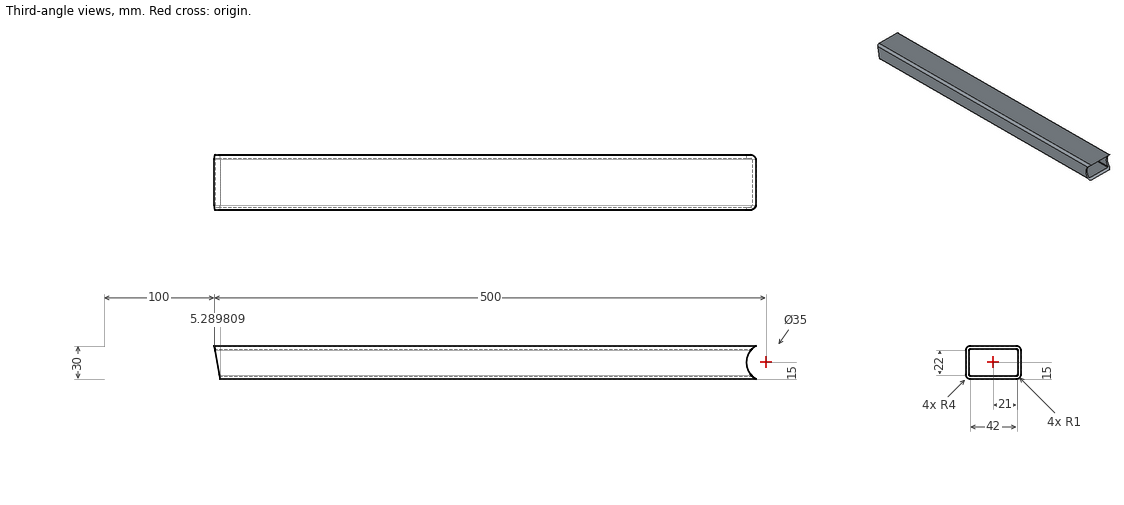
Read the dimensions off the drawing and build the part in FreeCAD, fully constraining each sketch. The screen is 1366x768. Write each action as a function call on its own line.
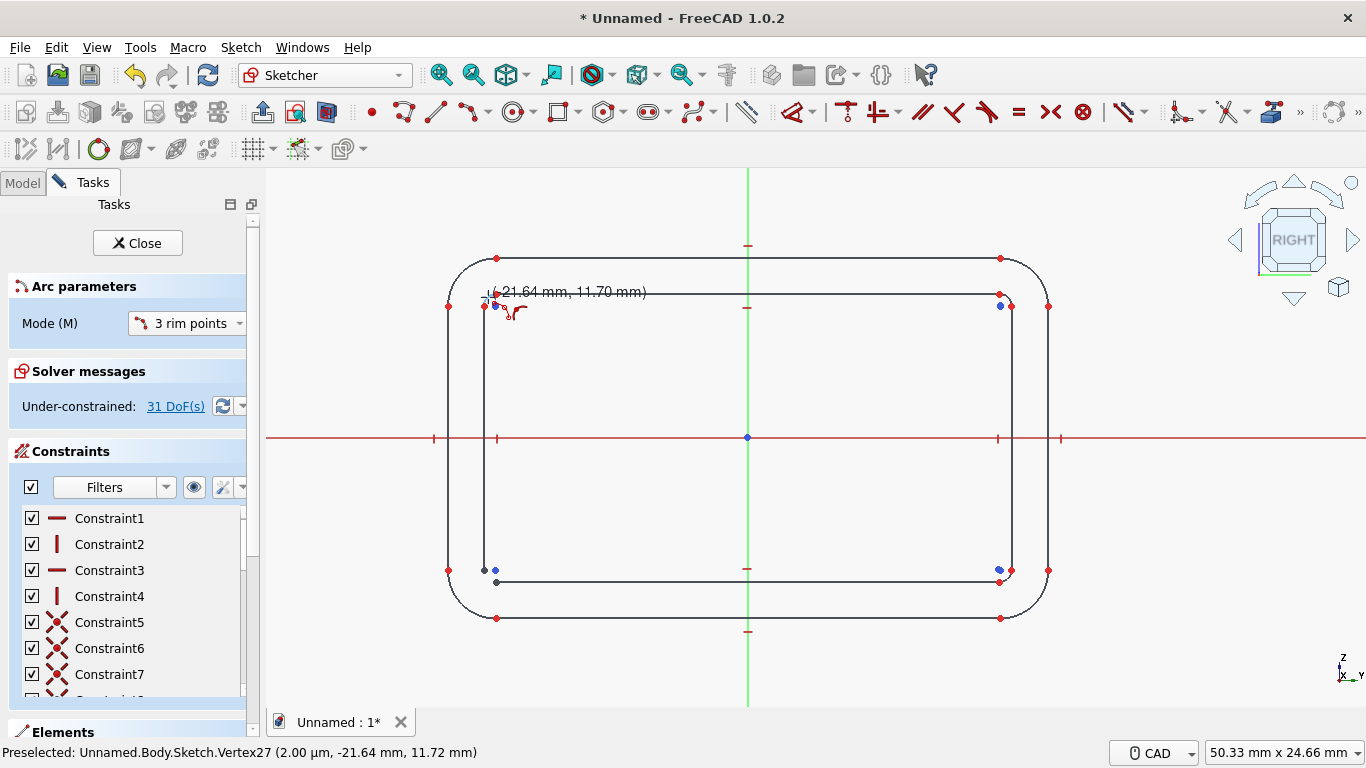
scroll(484, 570, up, 2)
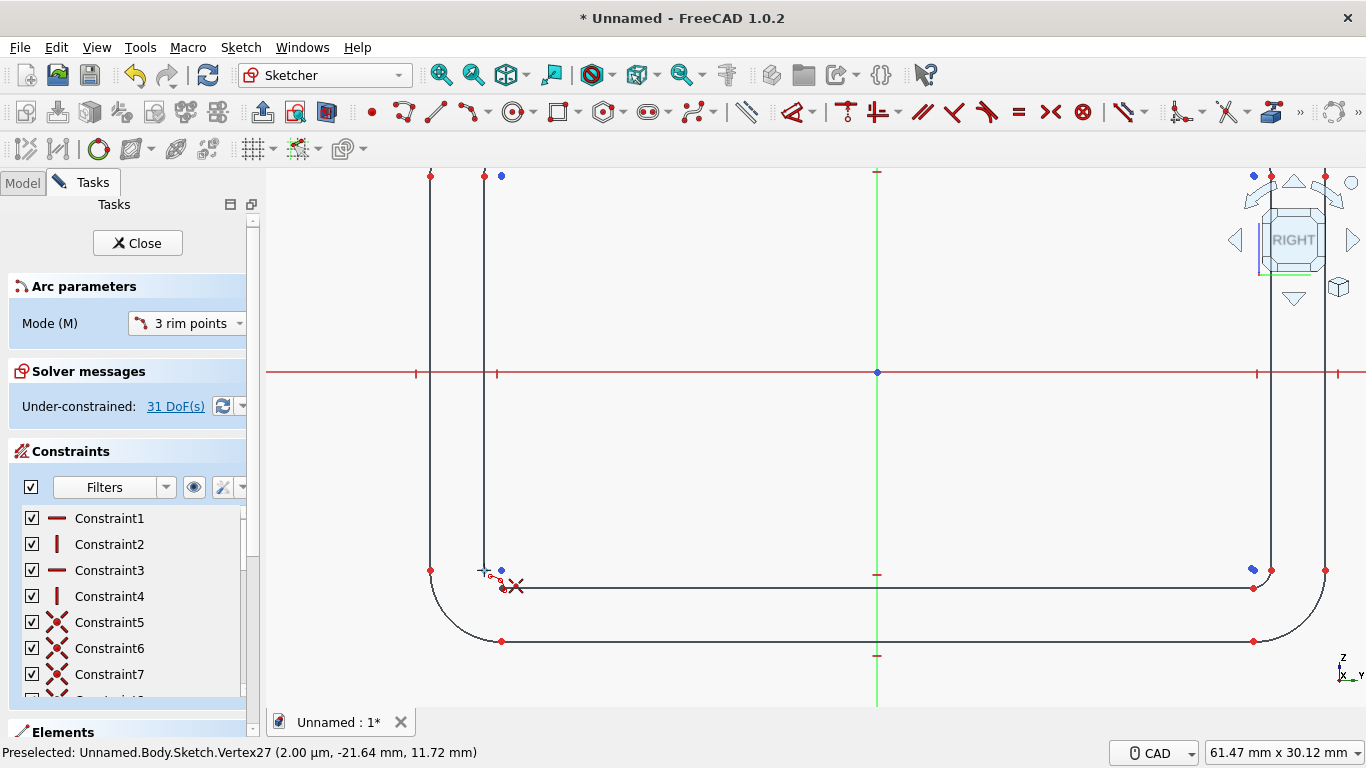
click(484, 570)
click(502, 588)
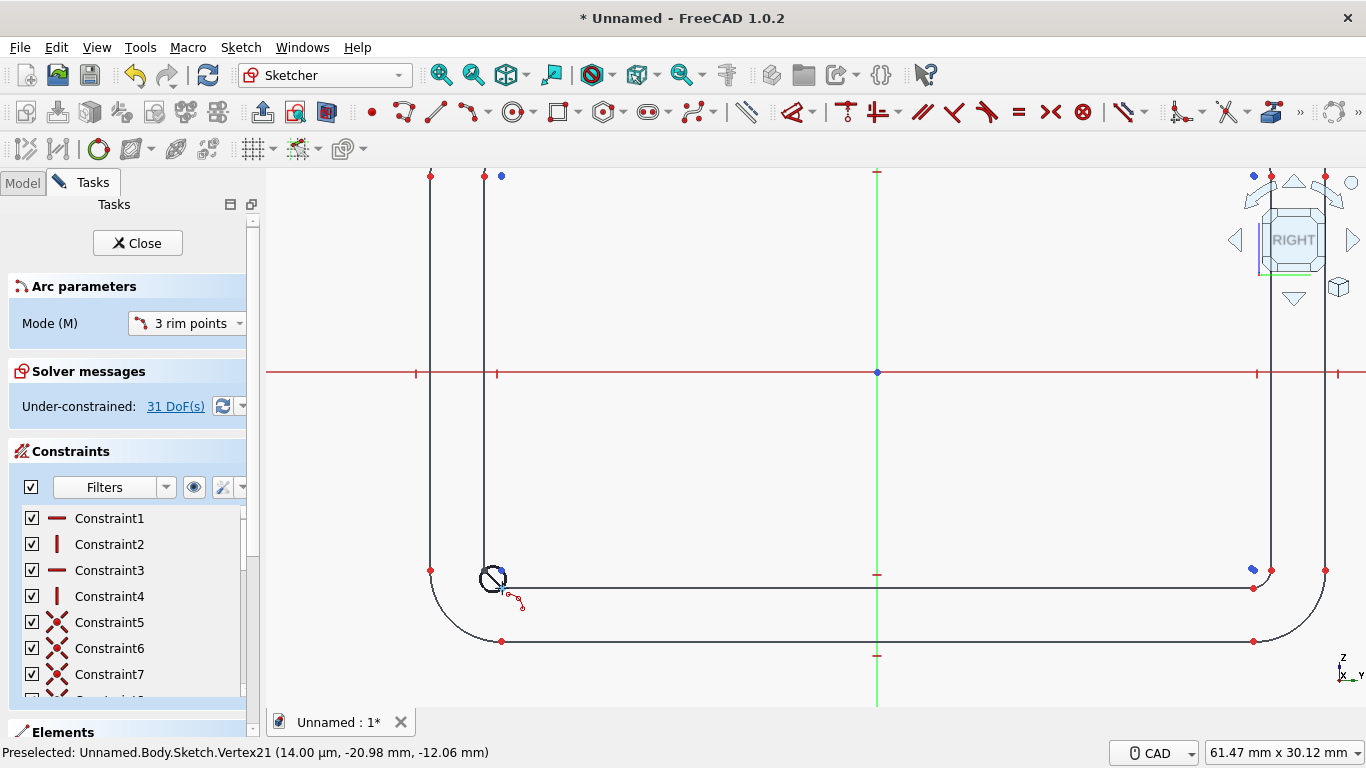
scroll(489, 582, up, 6)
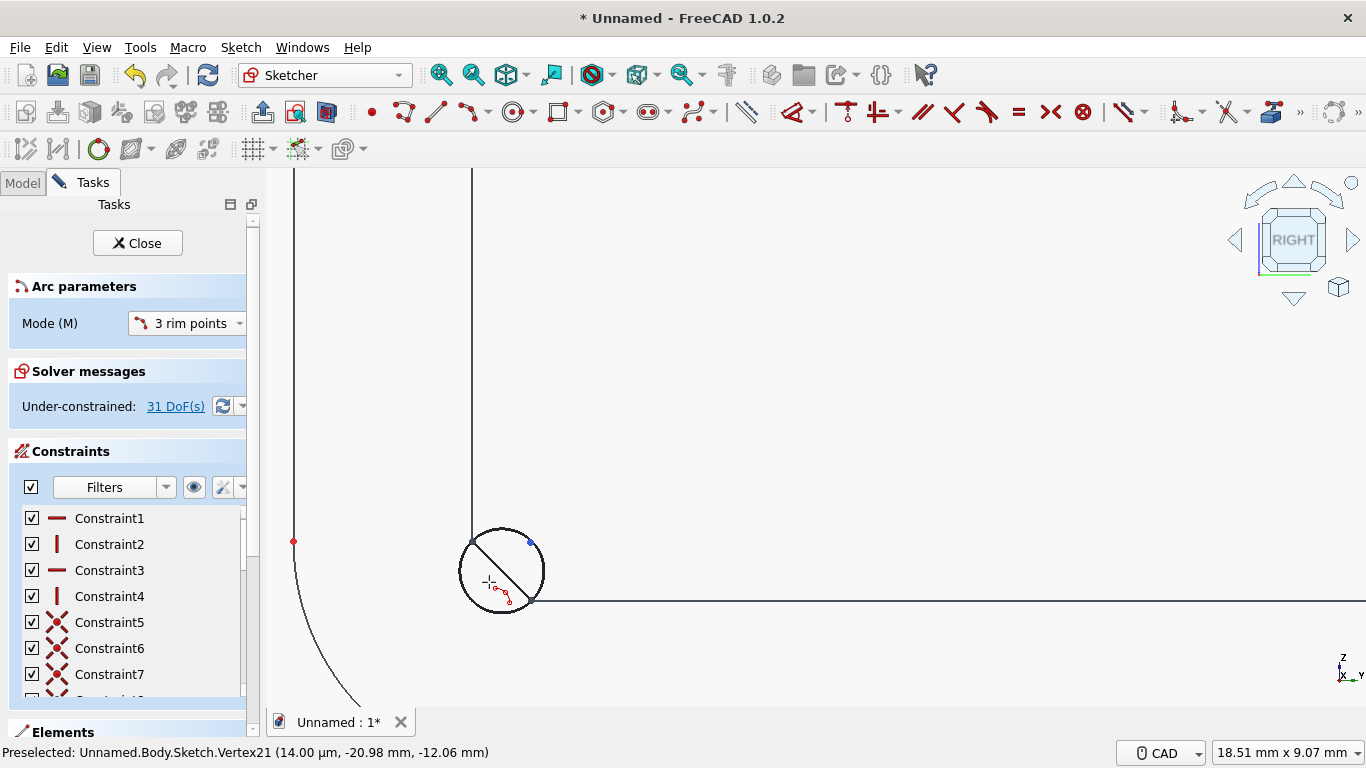
click(488, 580)
key(Escape)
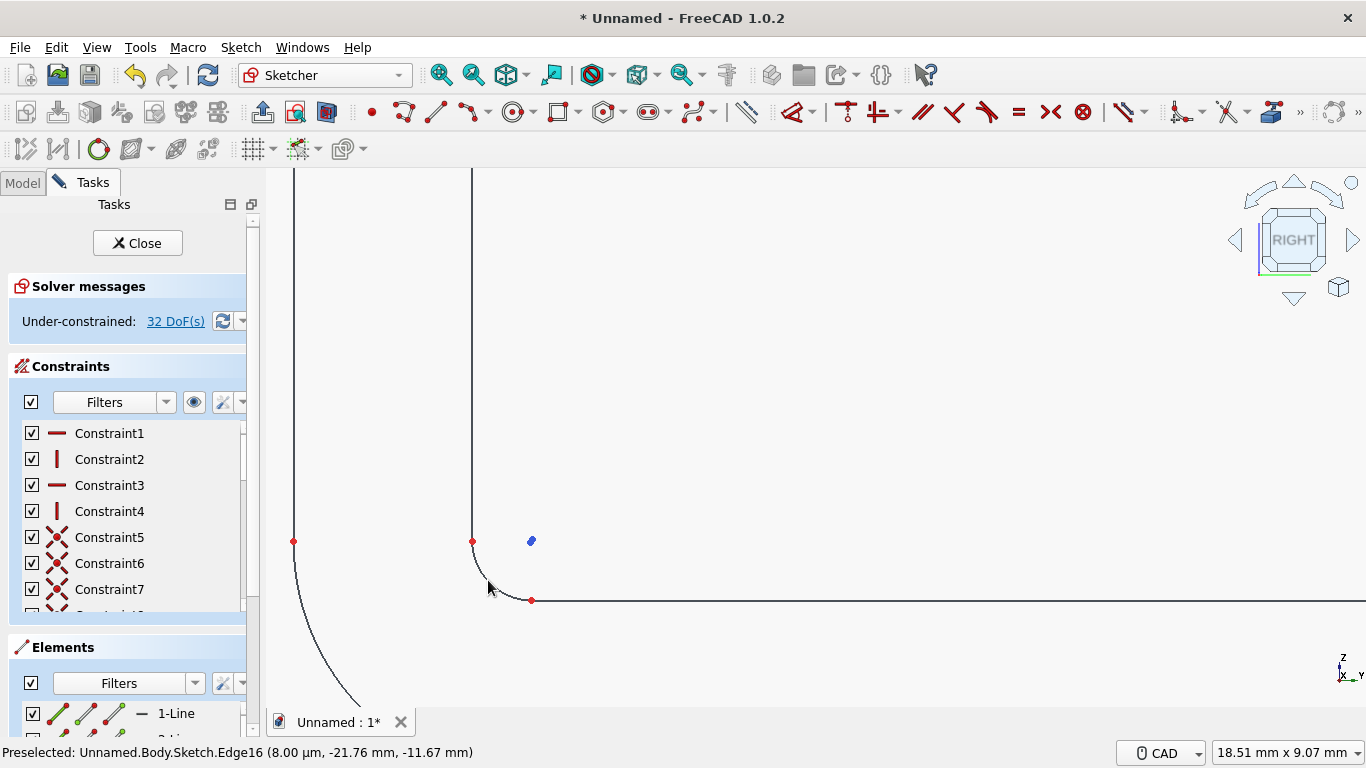
scroll(487, 577, down, 8)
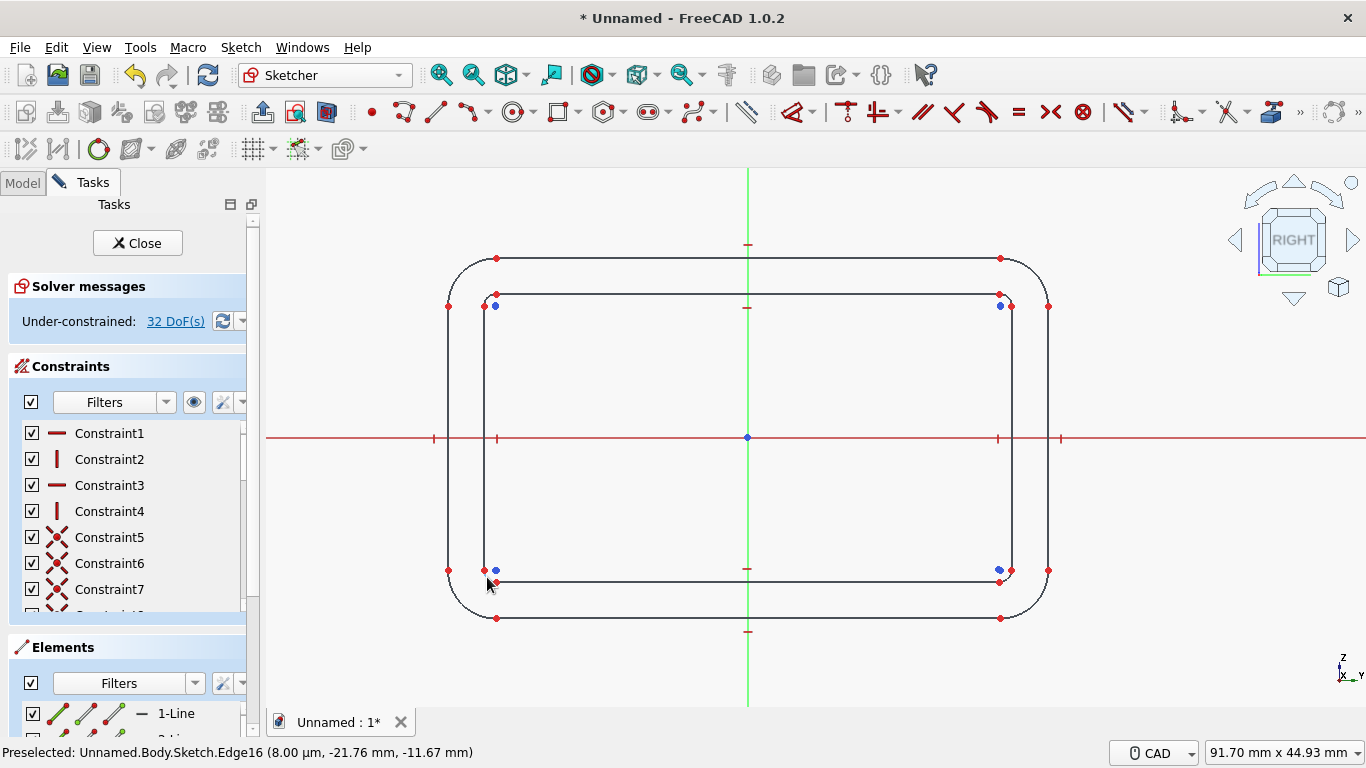
click(849, 618)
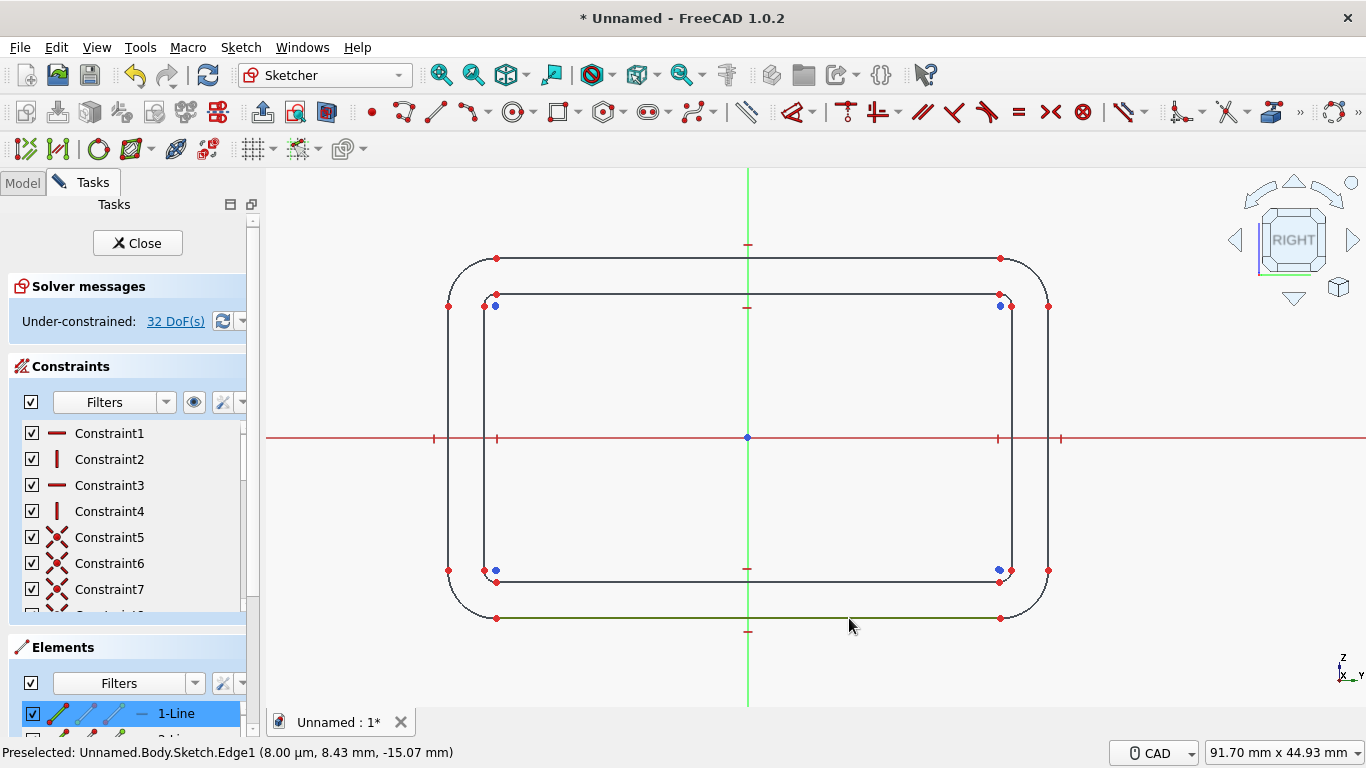
click(453, 592)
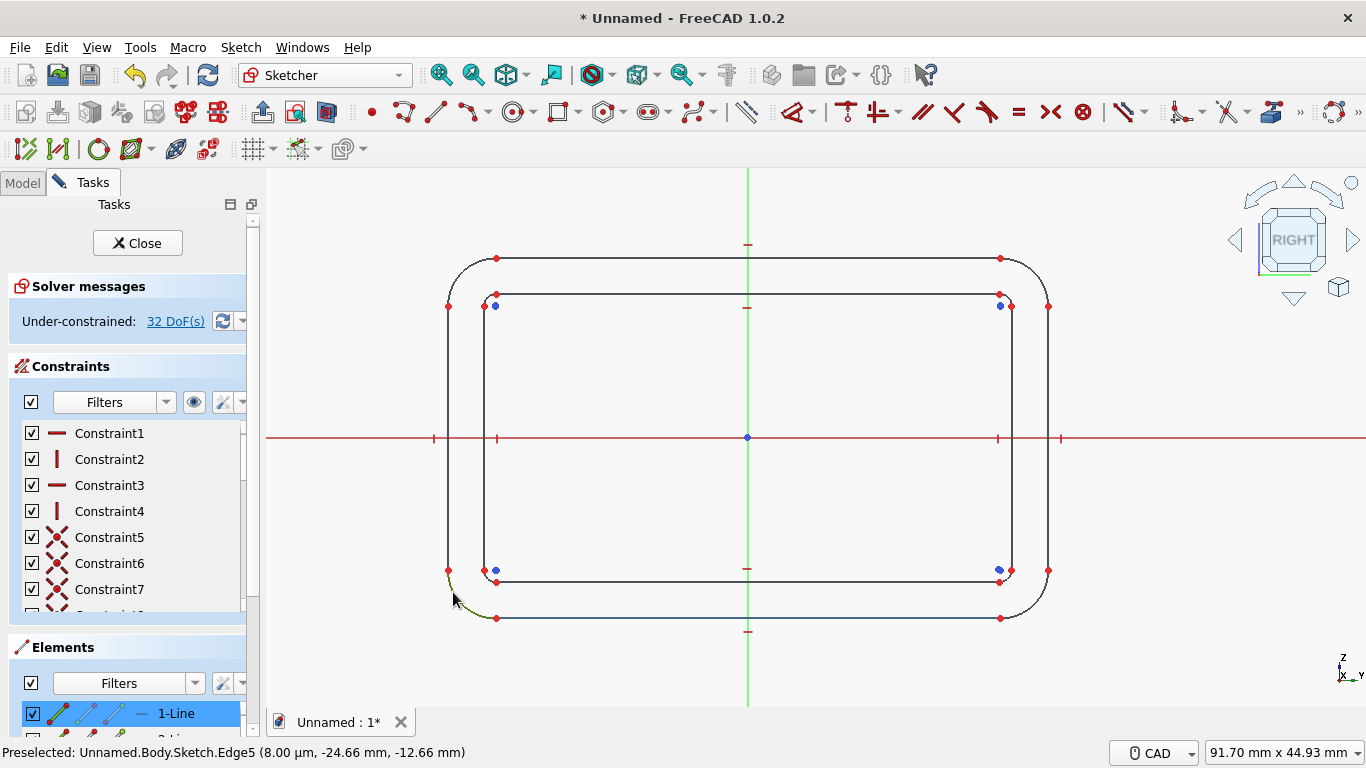
key(t)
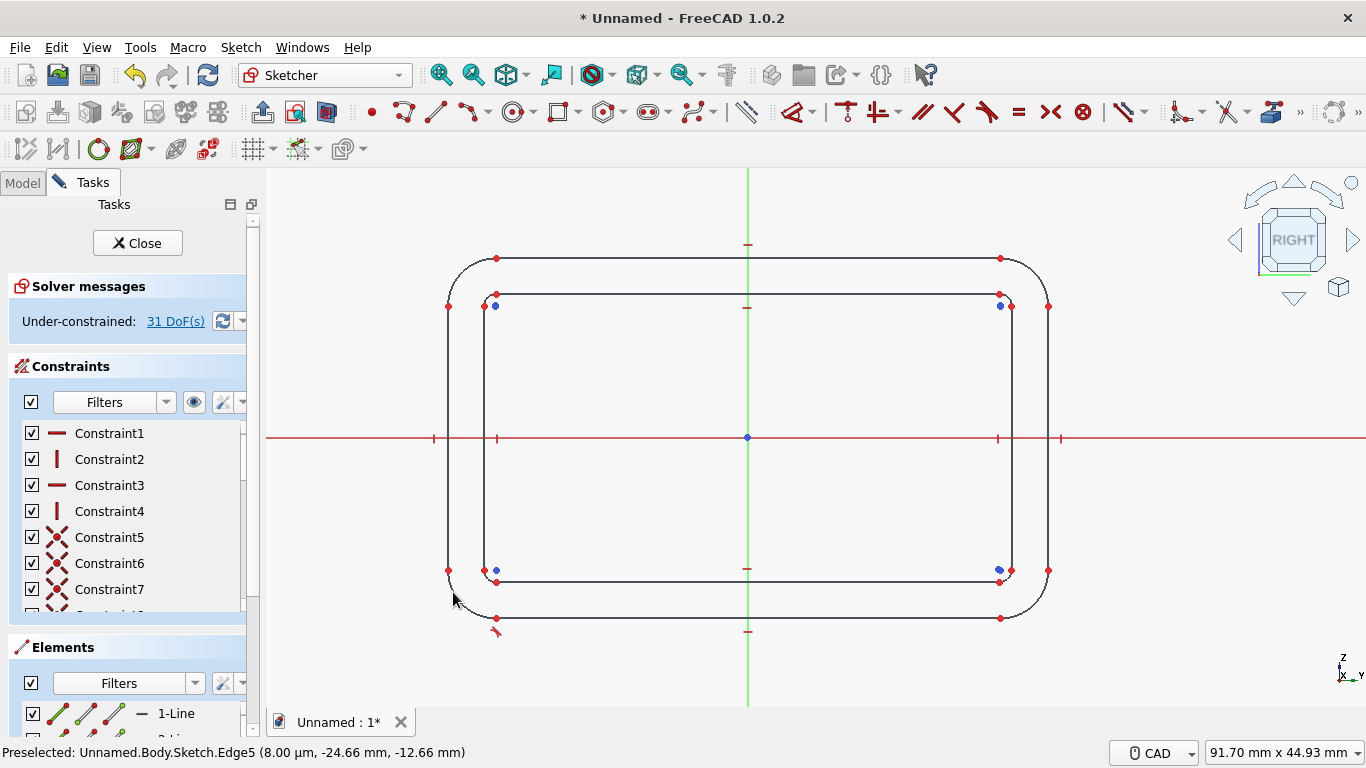
click(849, 618)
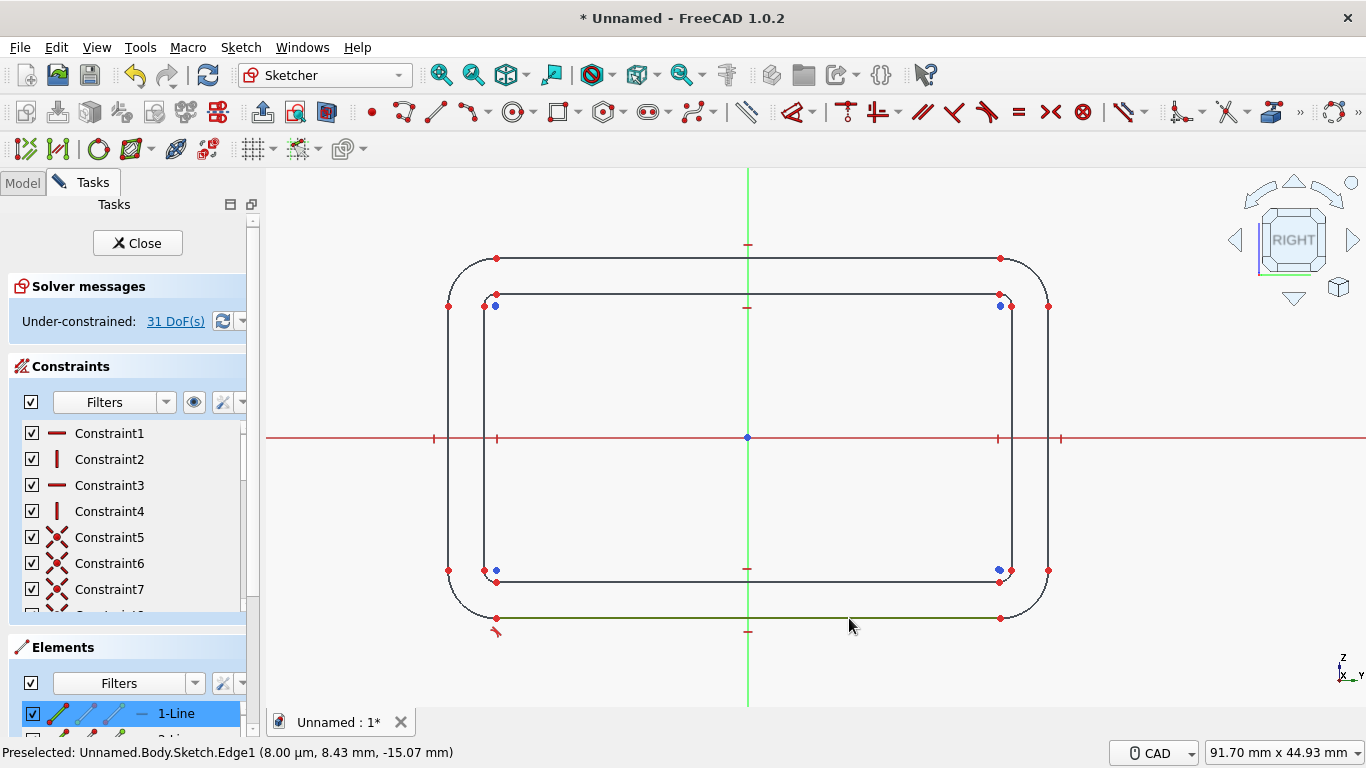
click(1022, 613)